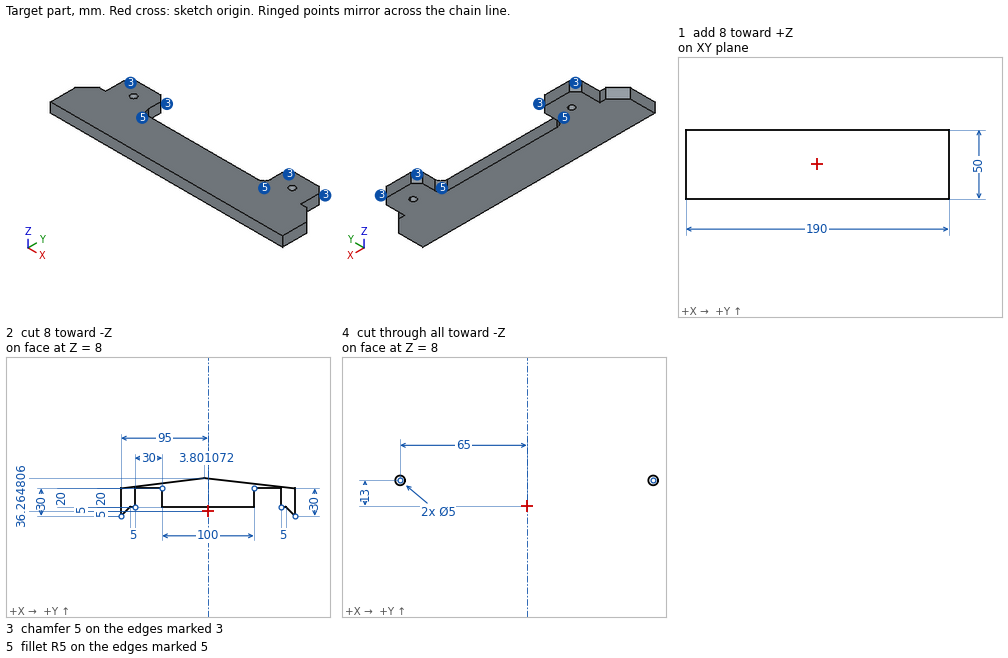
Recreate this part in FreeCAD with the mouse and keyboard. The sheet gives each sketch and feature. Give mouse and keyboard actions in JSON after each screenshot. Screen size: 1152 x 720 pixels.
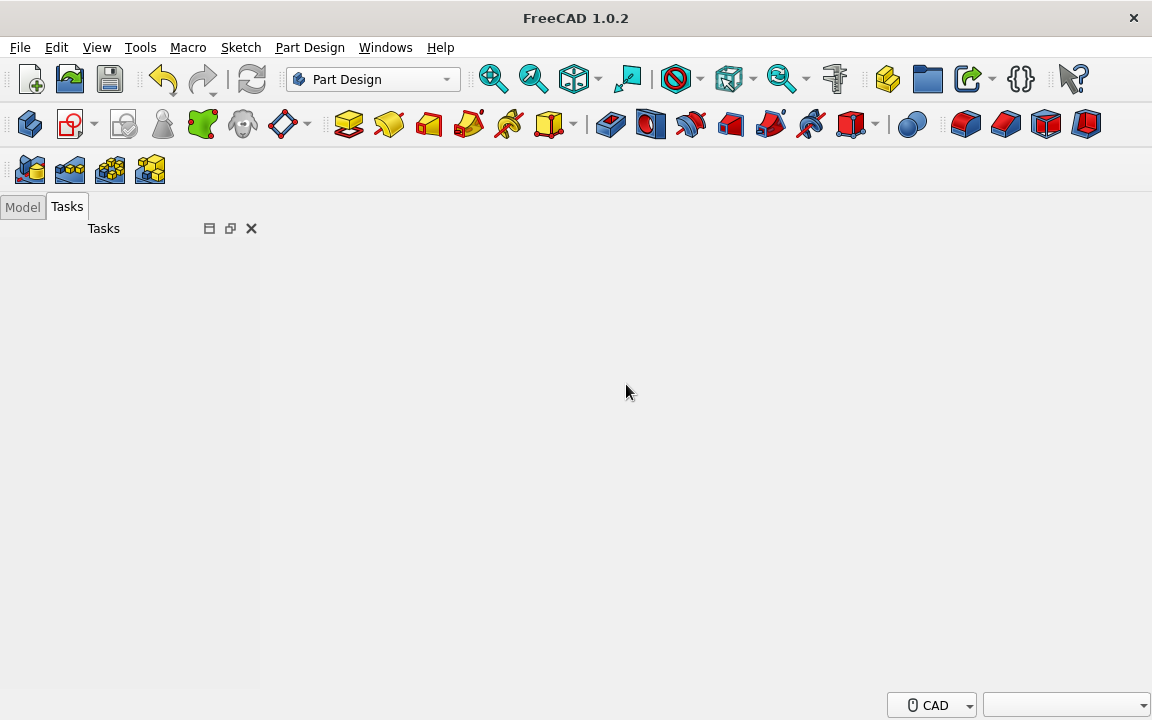
{"action": "key", "text": "ctrl+n"}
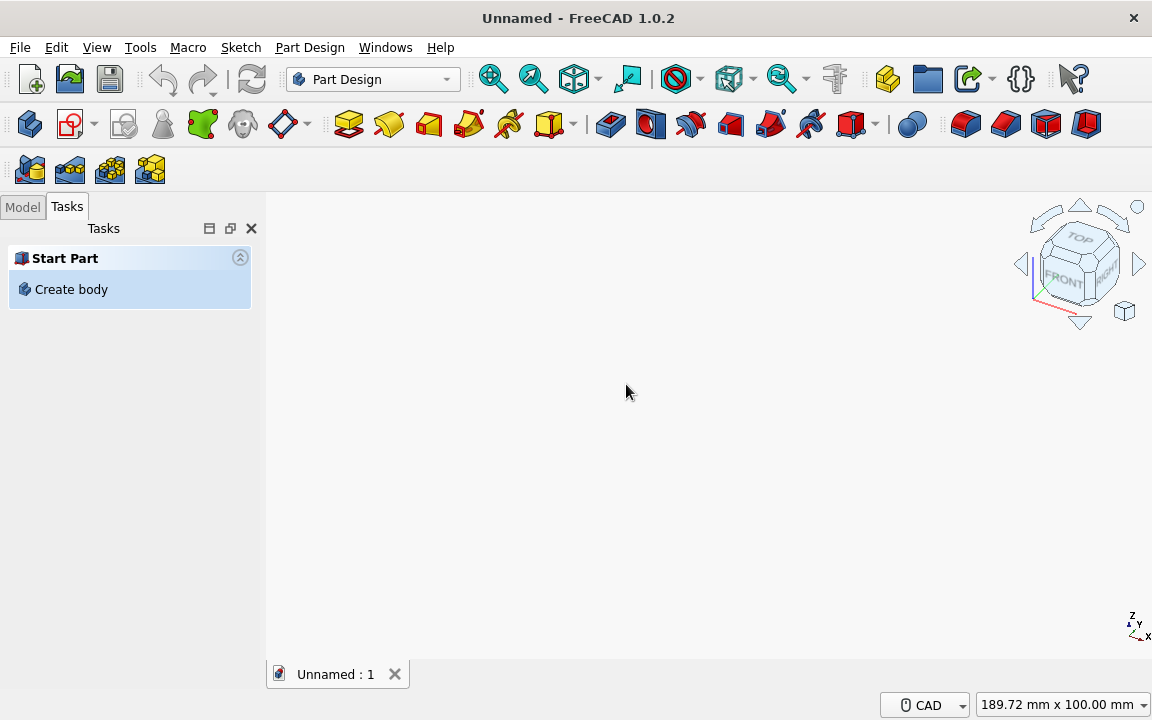
{"action": "left_click", "coordinate": [70, 124]}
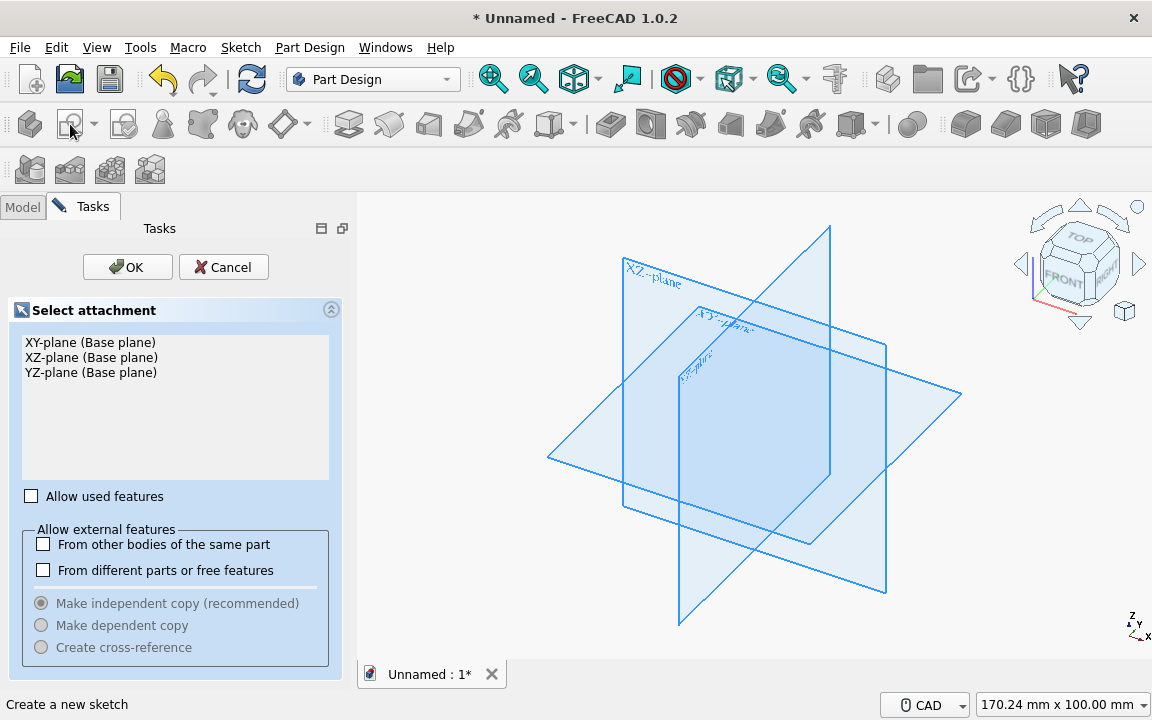
{"action": "left_click", "coordinate": [82, 342]}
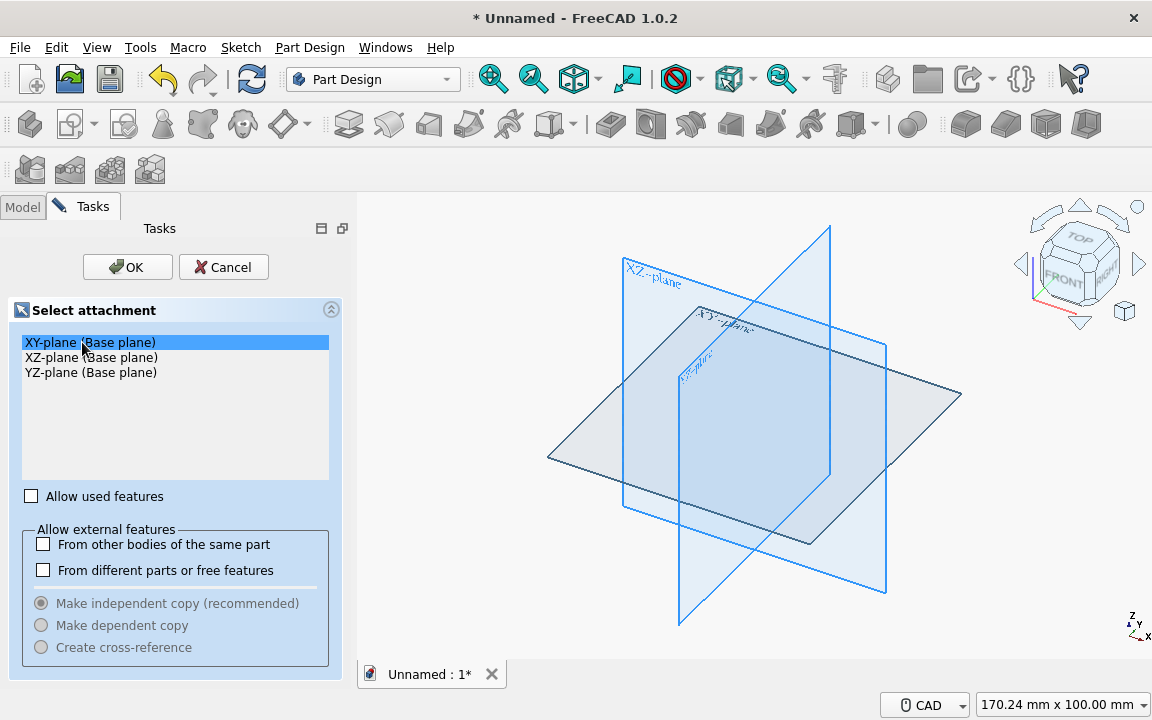
{"action": "left_click", "coordinate": [128, 267]}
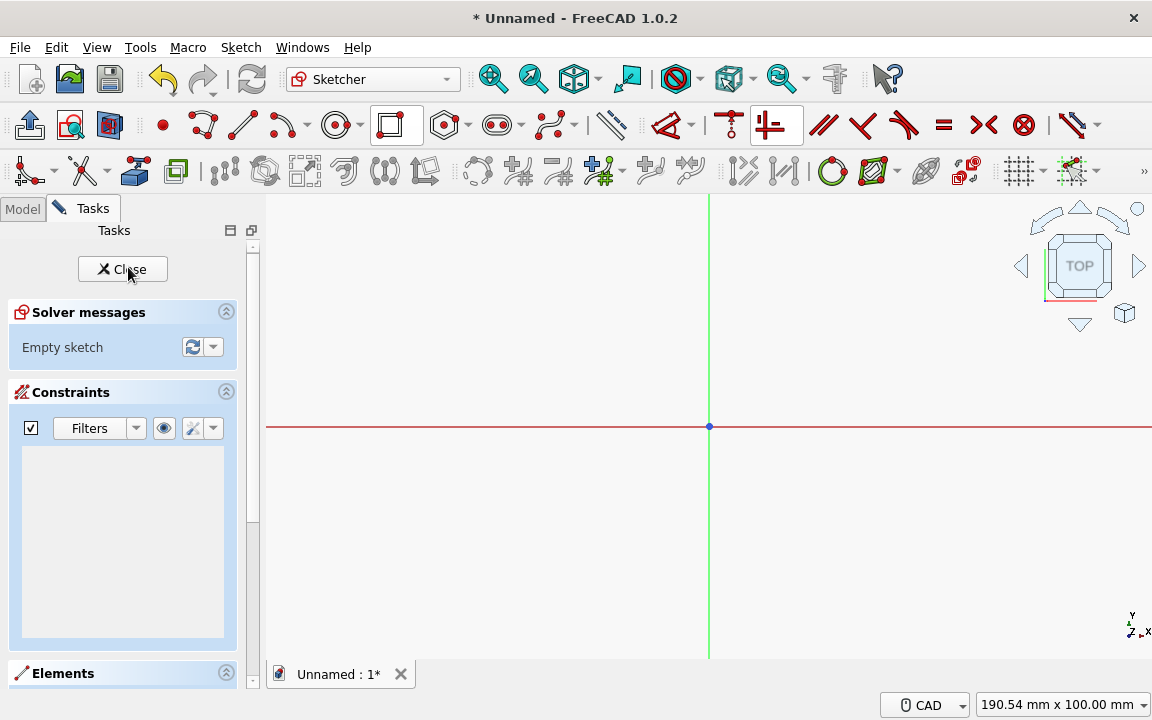
{"action": "scroll", "coordinate": [557, 426], "scroll_direction": "down", "scroll_amount": 3}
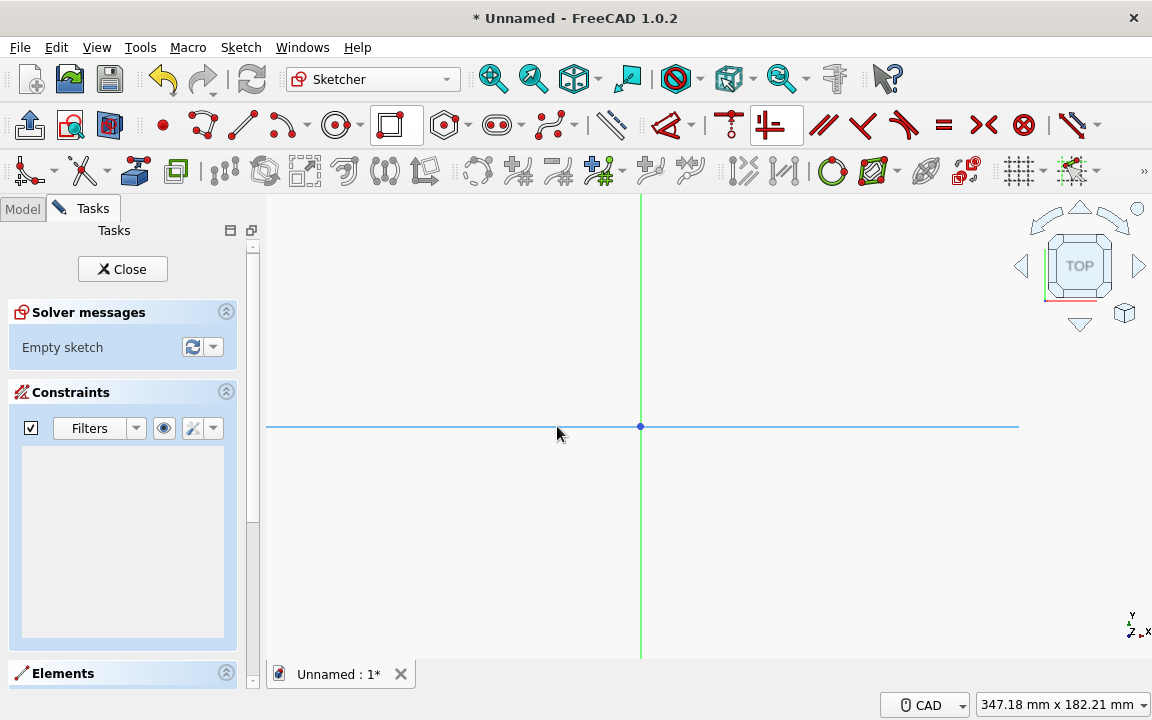
{"action": "key", "text": "g v"}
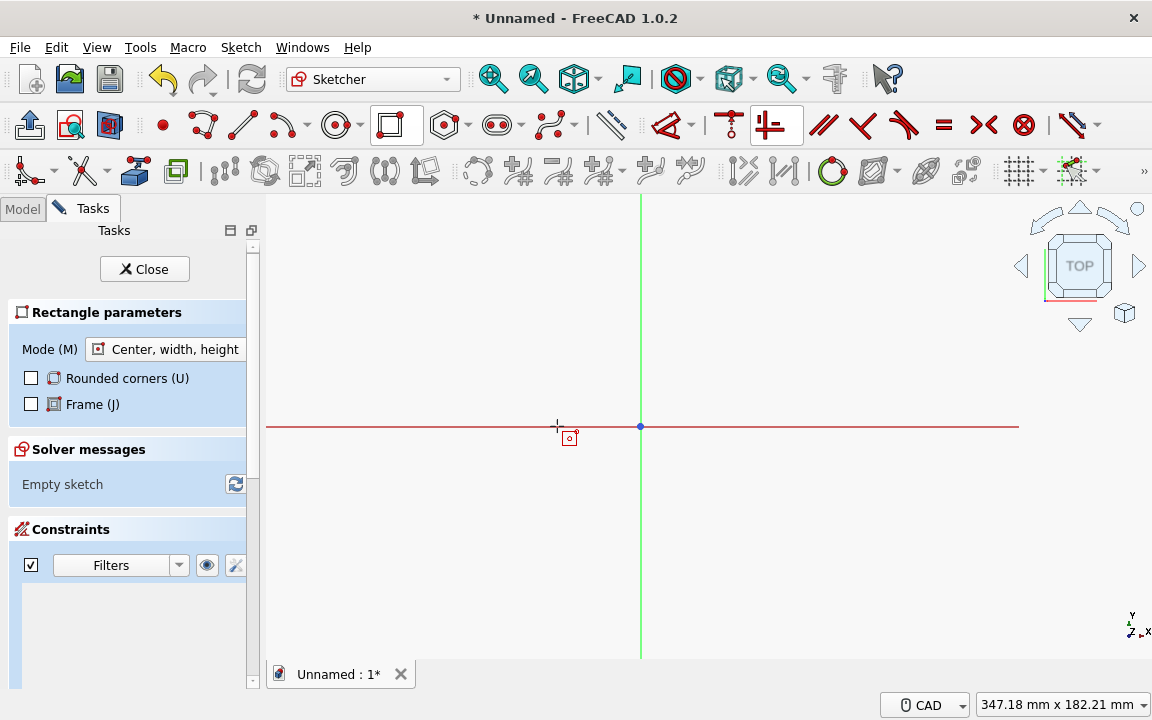
{"action": "left_click", "coordinate": [641, 426]}
{"action": "mouse_move", "coordinate": [883, 363]}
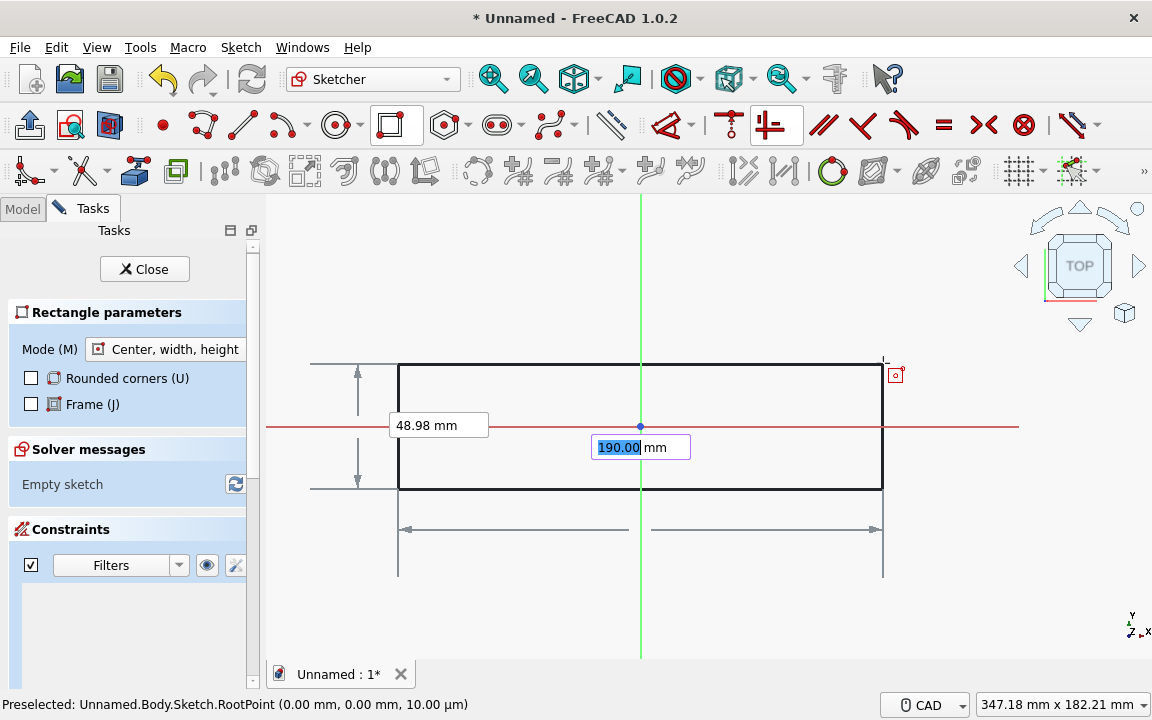
{"action": "type", "text": "190"}
{"action": "key", "text": "Tab"}
{"action": "type", "text": "50"}
{"action": "key", "text": "Return"}
{"action": "key", "text": "Escape"}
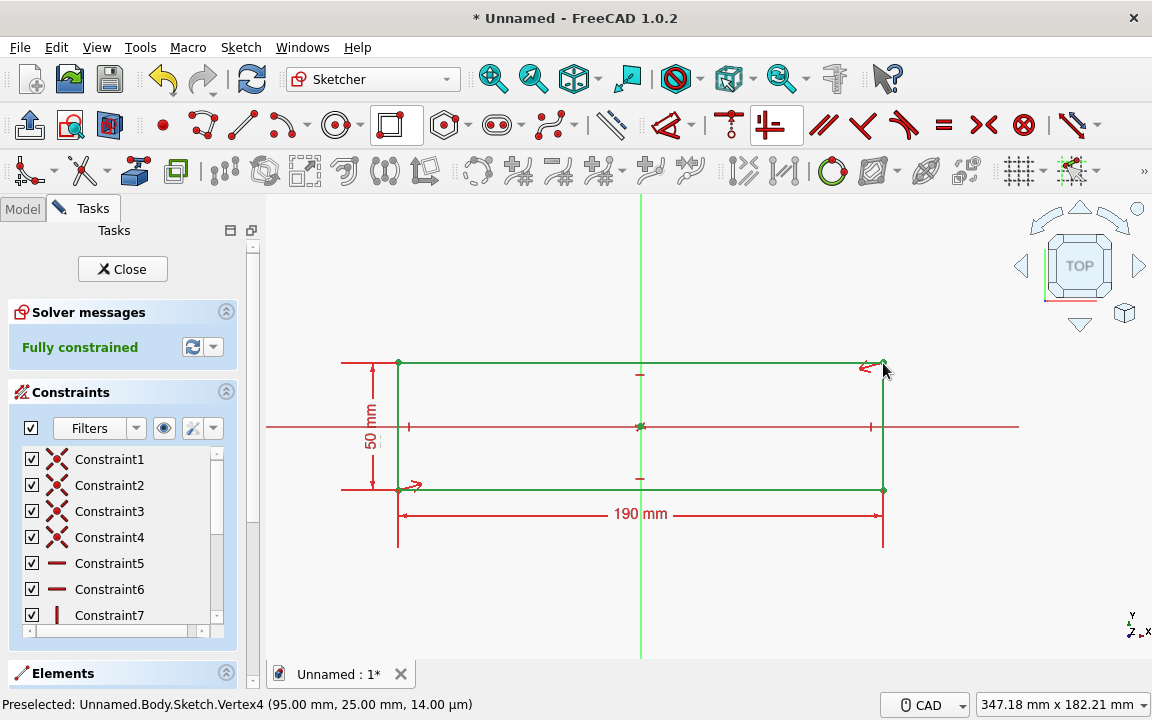
{"action": "left_click", "coordinate": [123, 269]}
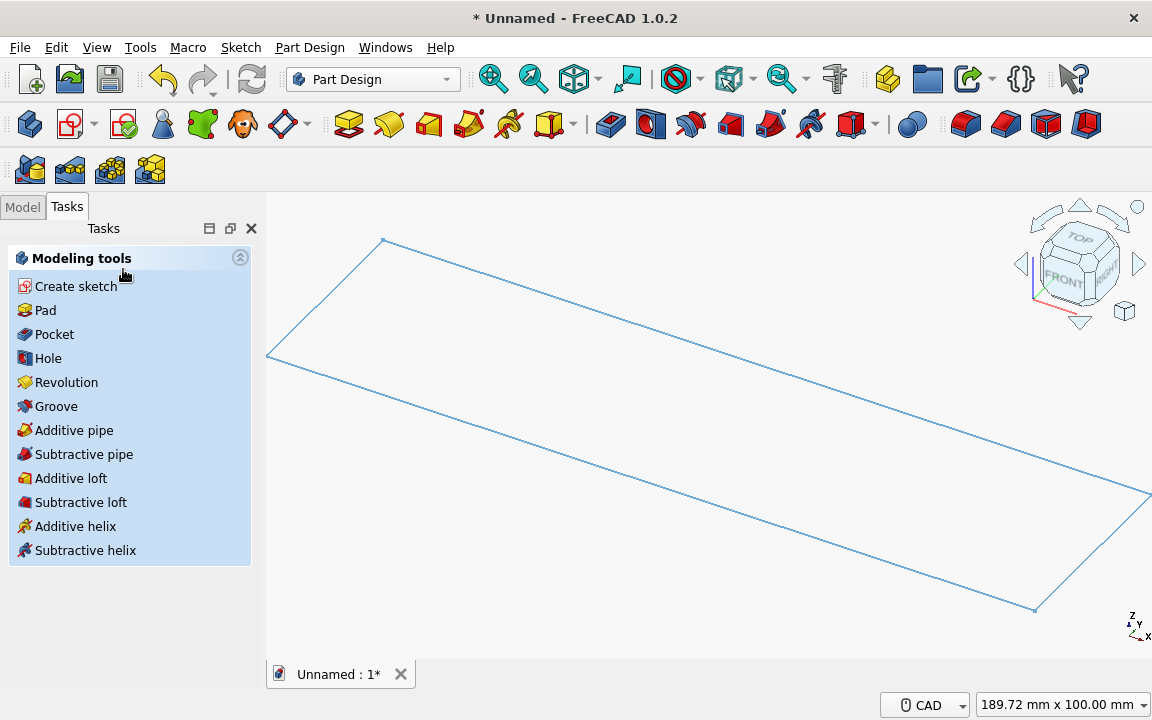
{"action": "left_click", "coordinate": [350, 124]}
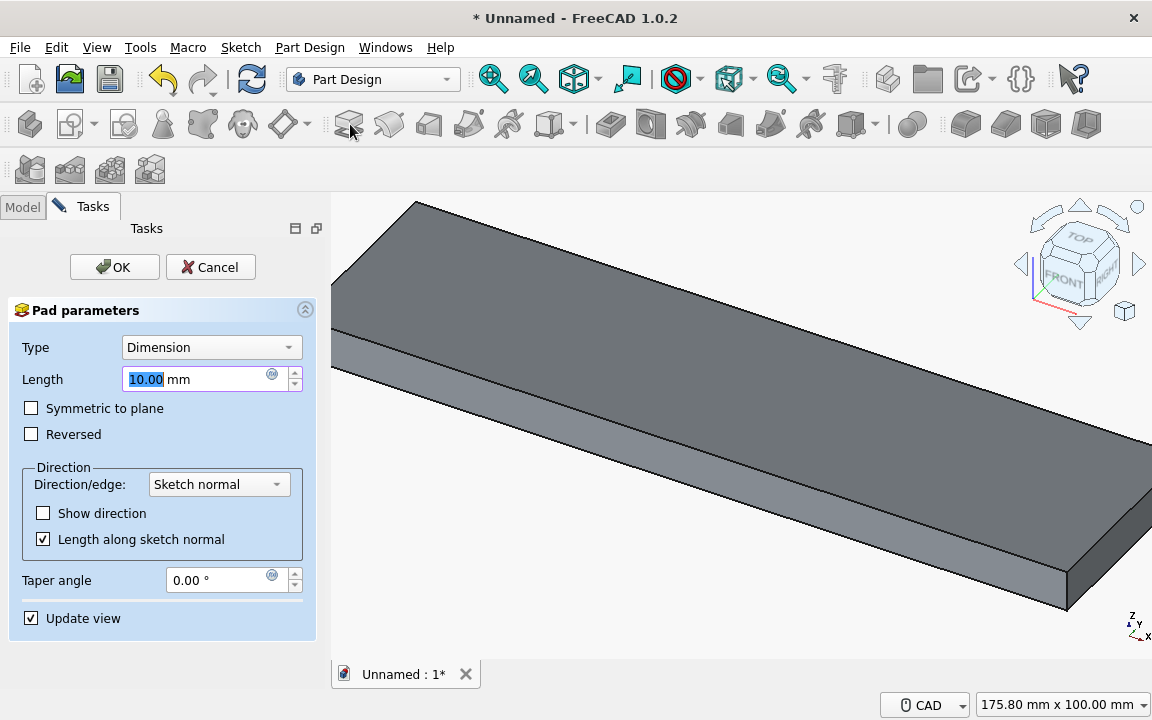
{"action": "type", "text": "8"}
{"action": "key", "text": "Tab"}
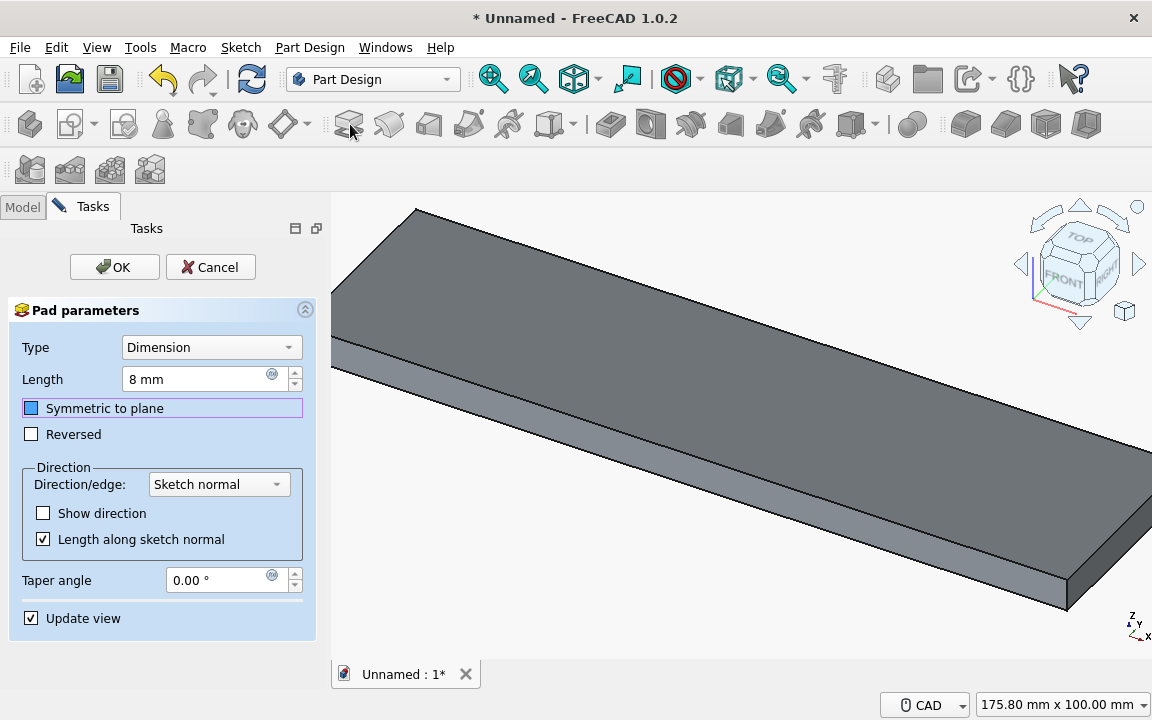
{"action": "left_click", "coordinate": [115, 267]}